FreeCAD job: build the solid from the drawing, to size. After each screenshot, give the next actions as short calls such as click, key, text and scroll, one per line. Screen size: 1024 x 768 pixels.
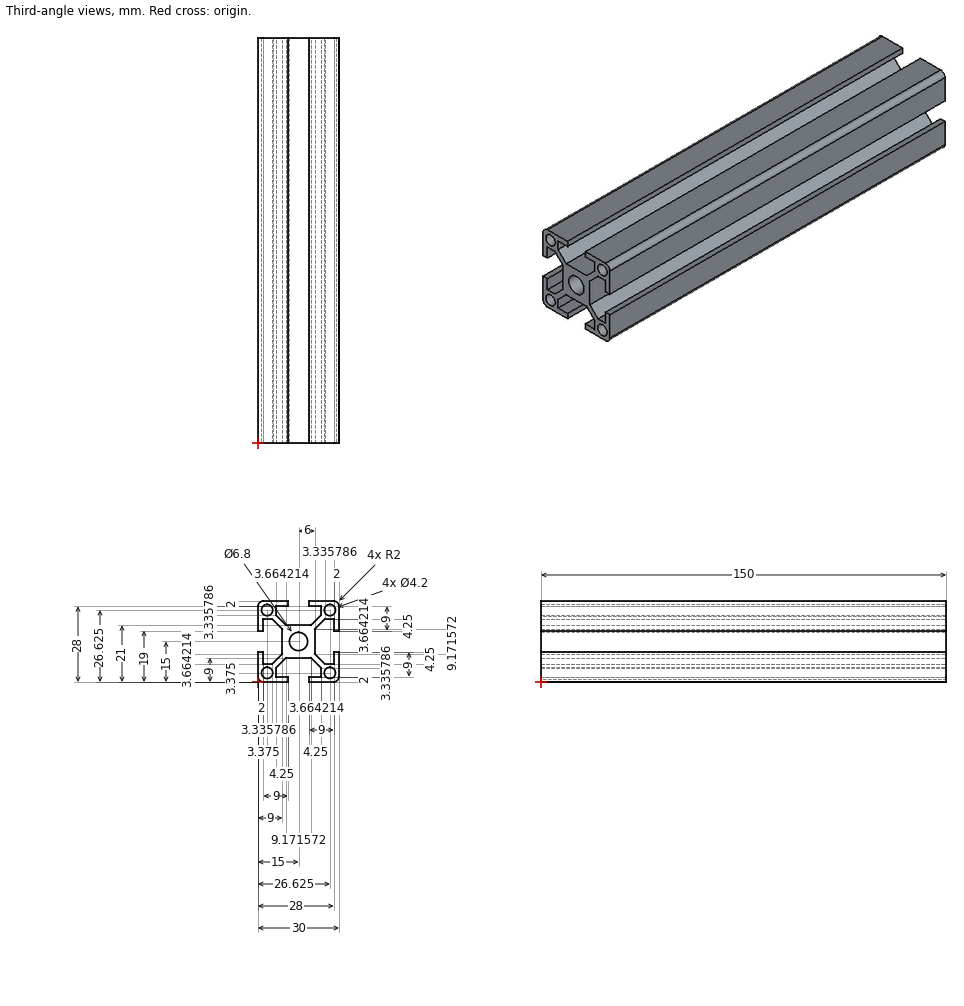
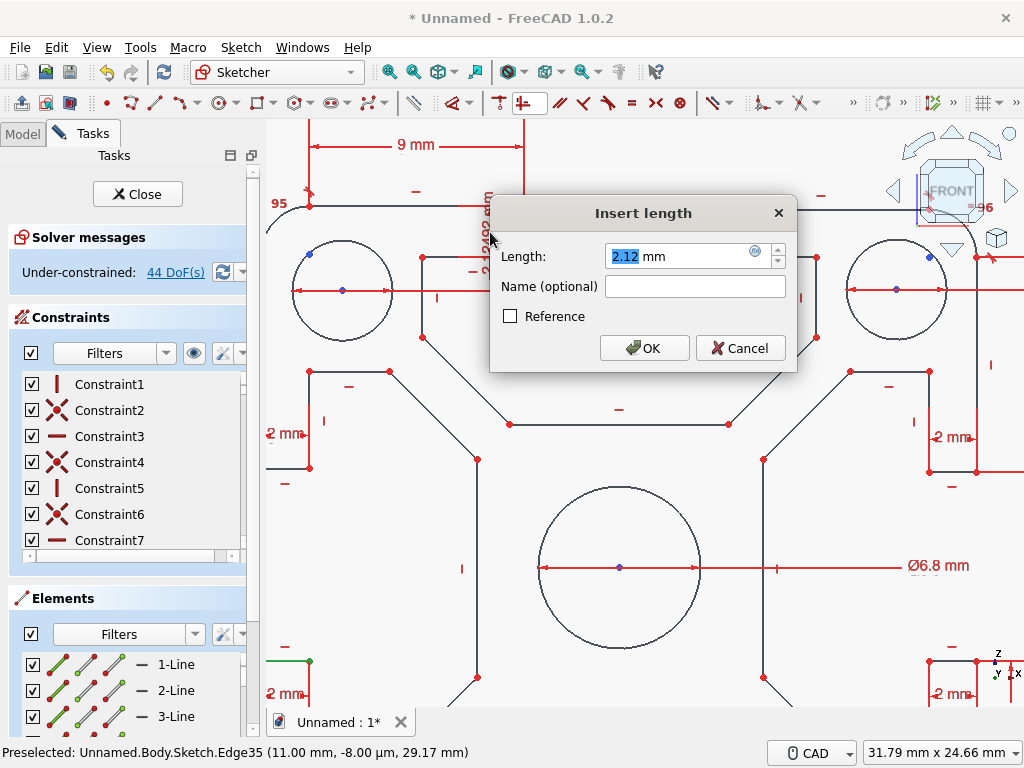
text(2)
key(Return)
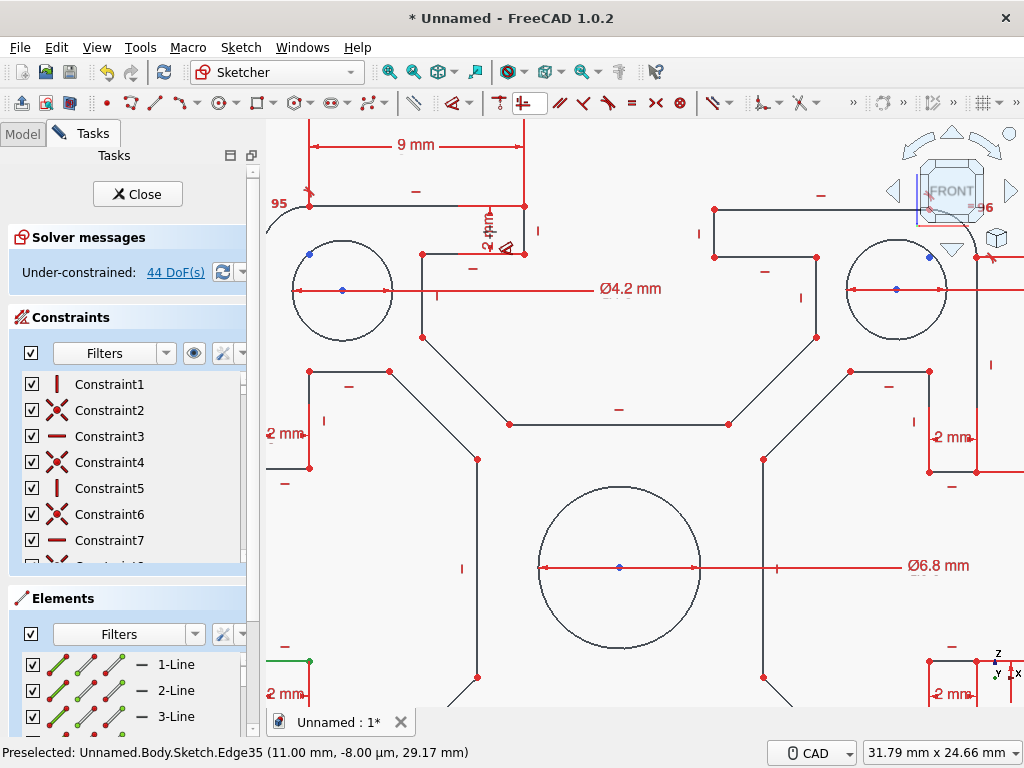
click(714, 243)
click(748, 233)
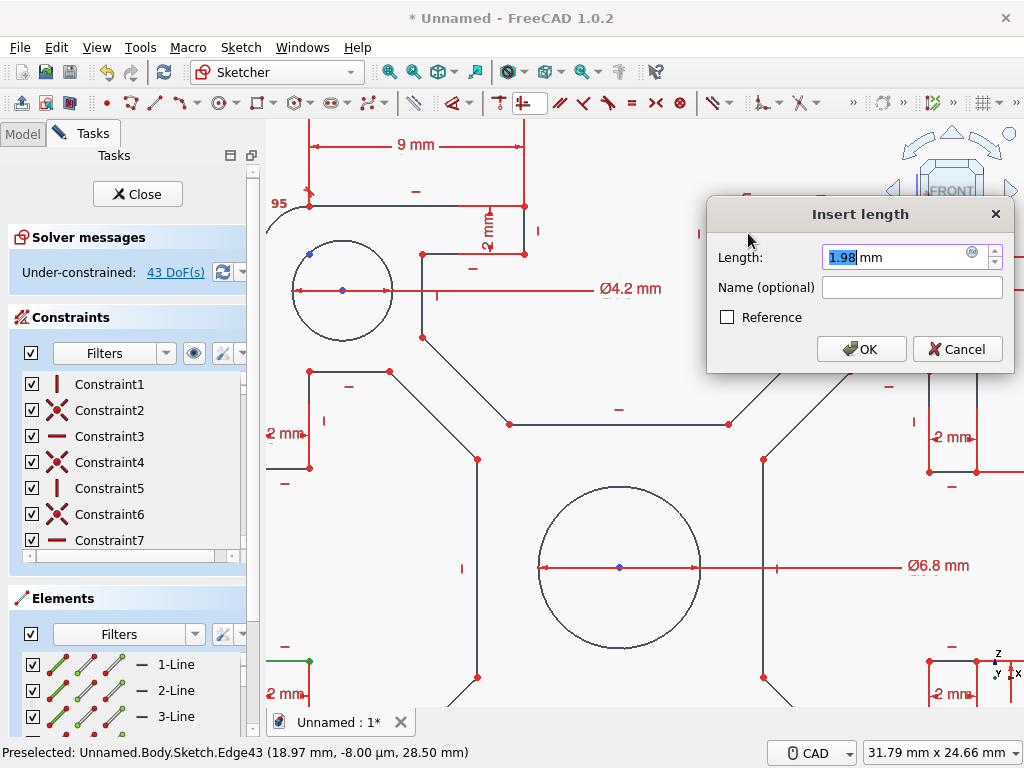
text(2)
key(Return)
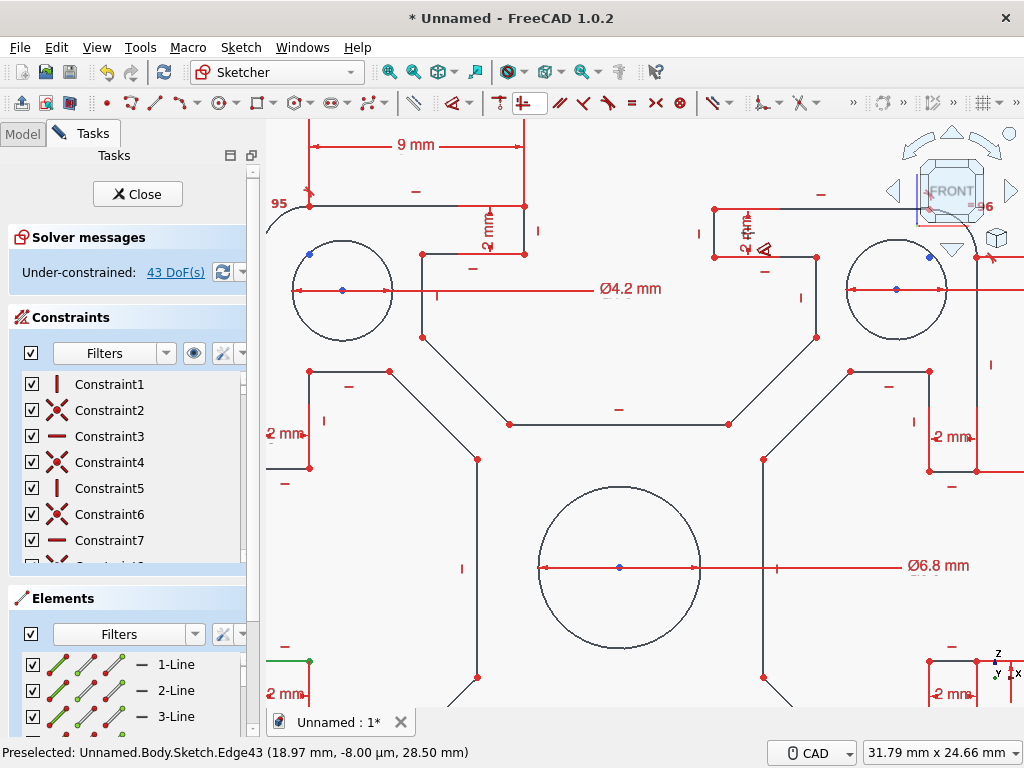
click(779, 209)
click(787, 175)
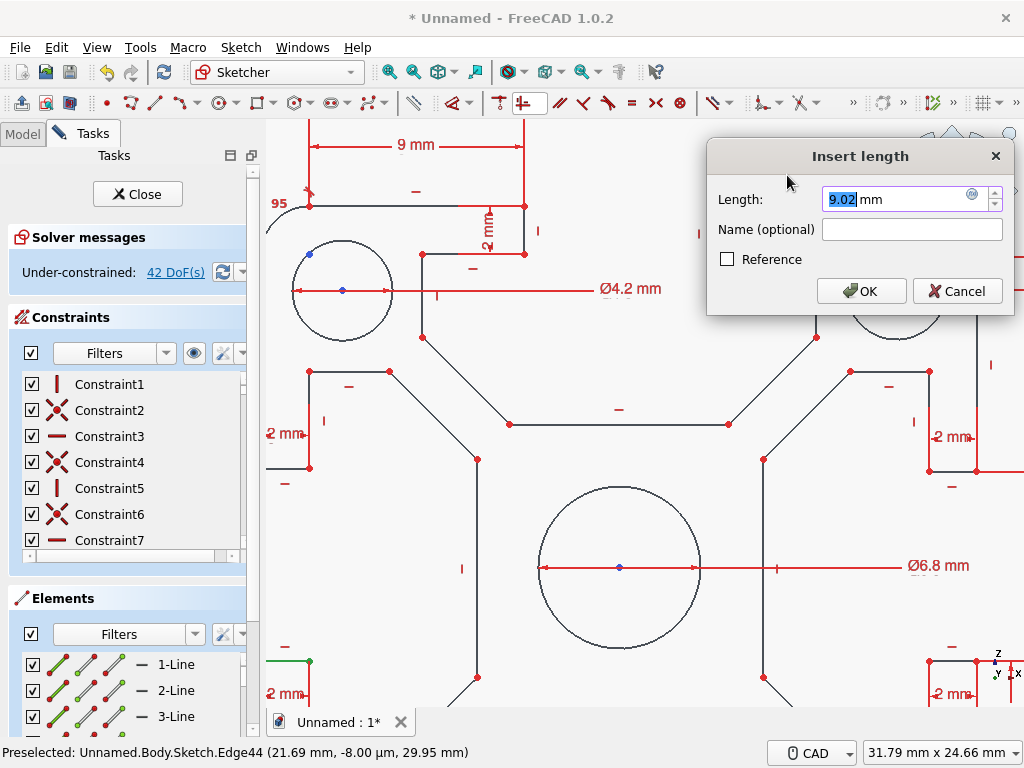
text(9)
key(Return)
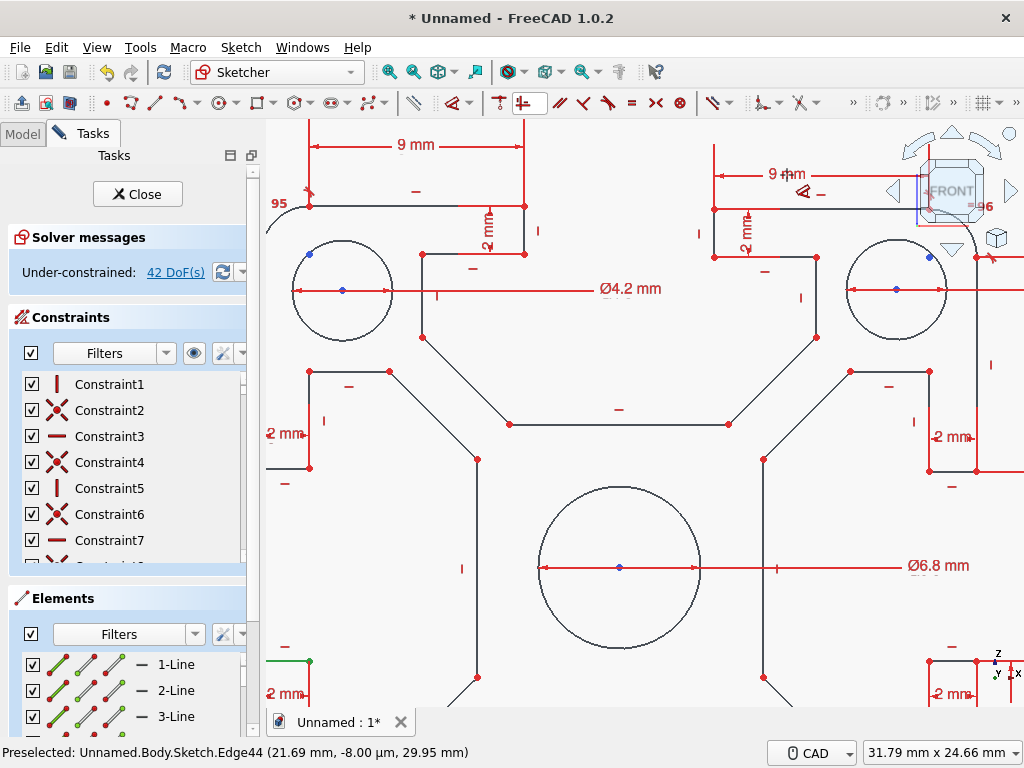
scroll(524, 227, down, 3)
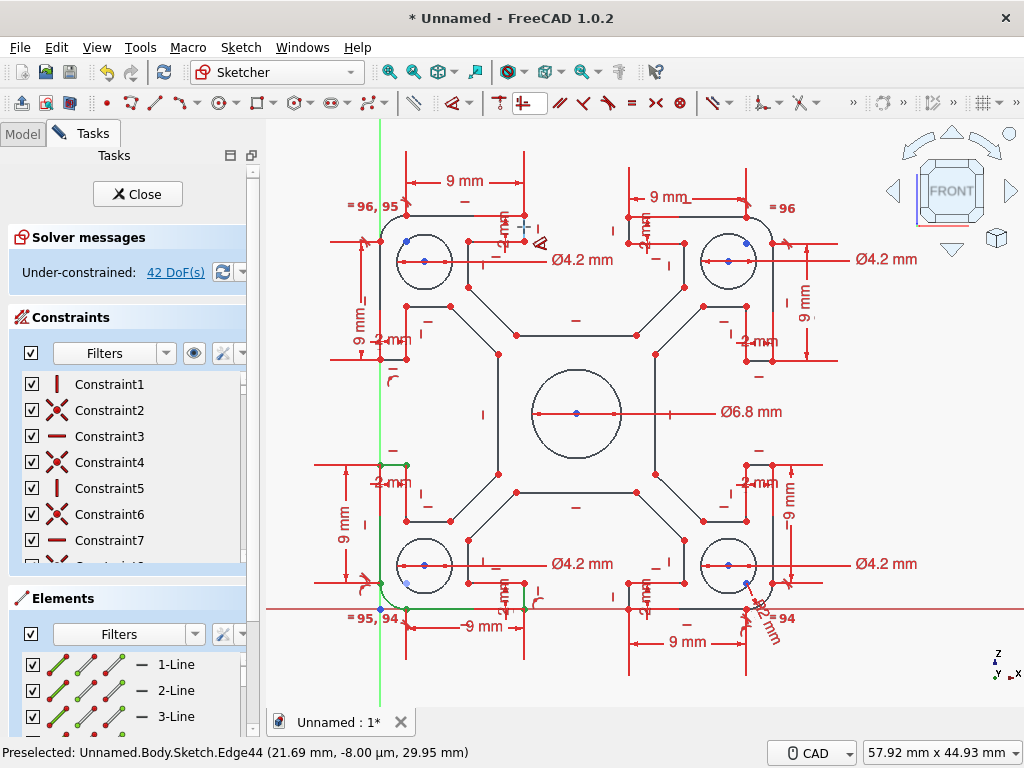
click(636, 493)
click(346, 551)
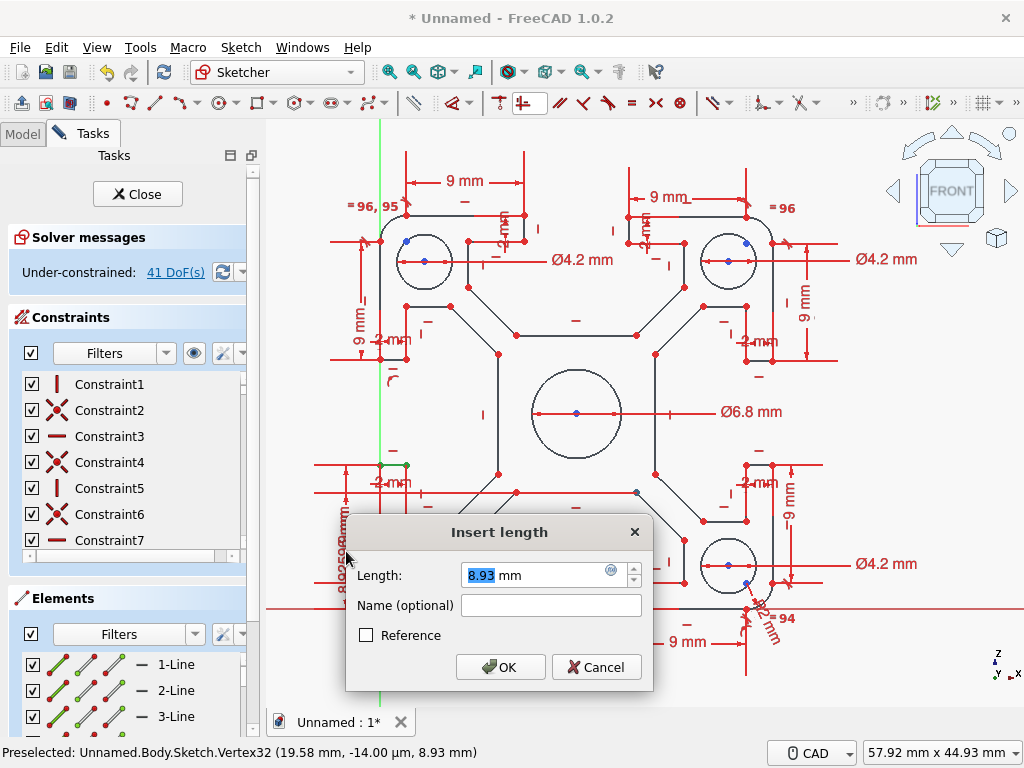
text(9)
key(Return)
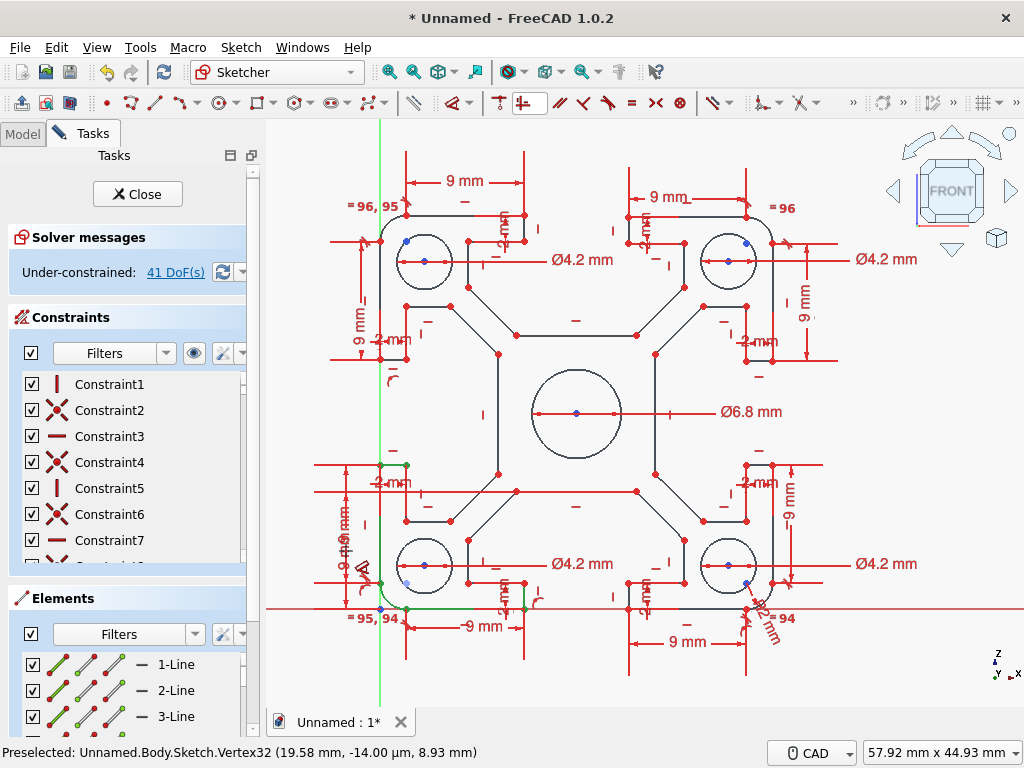
click(498, 475)
click(412, 643)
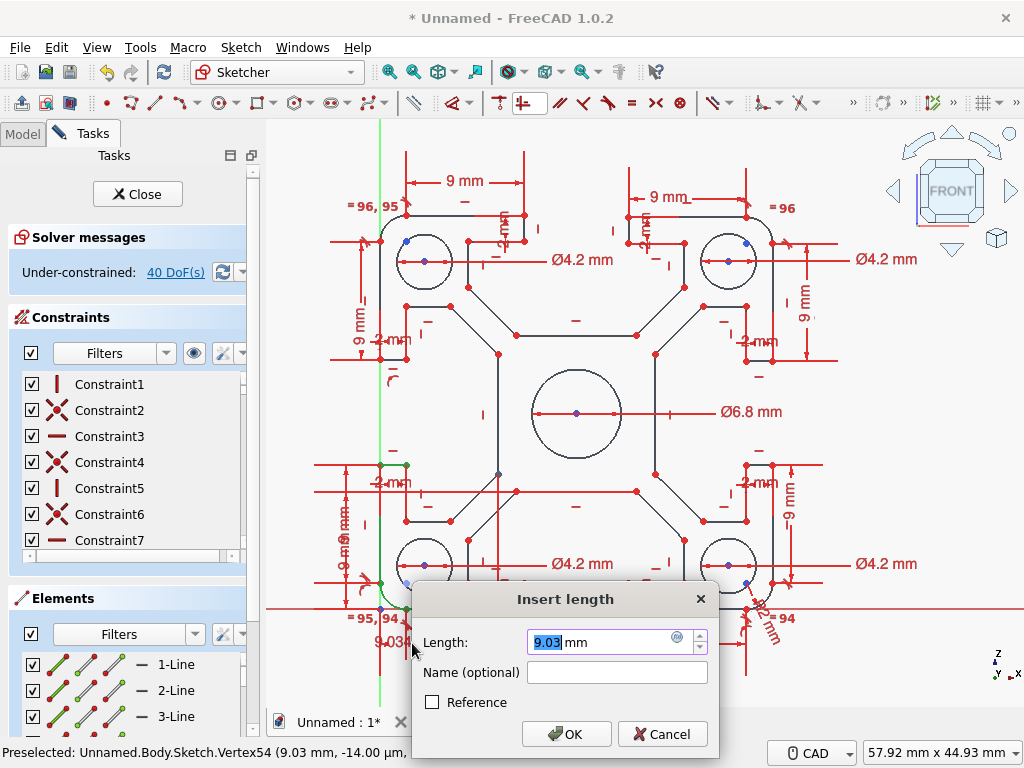
text(9)
key(Return)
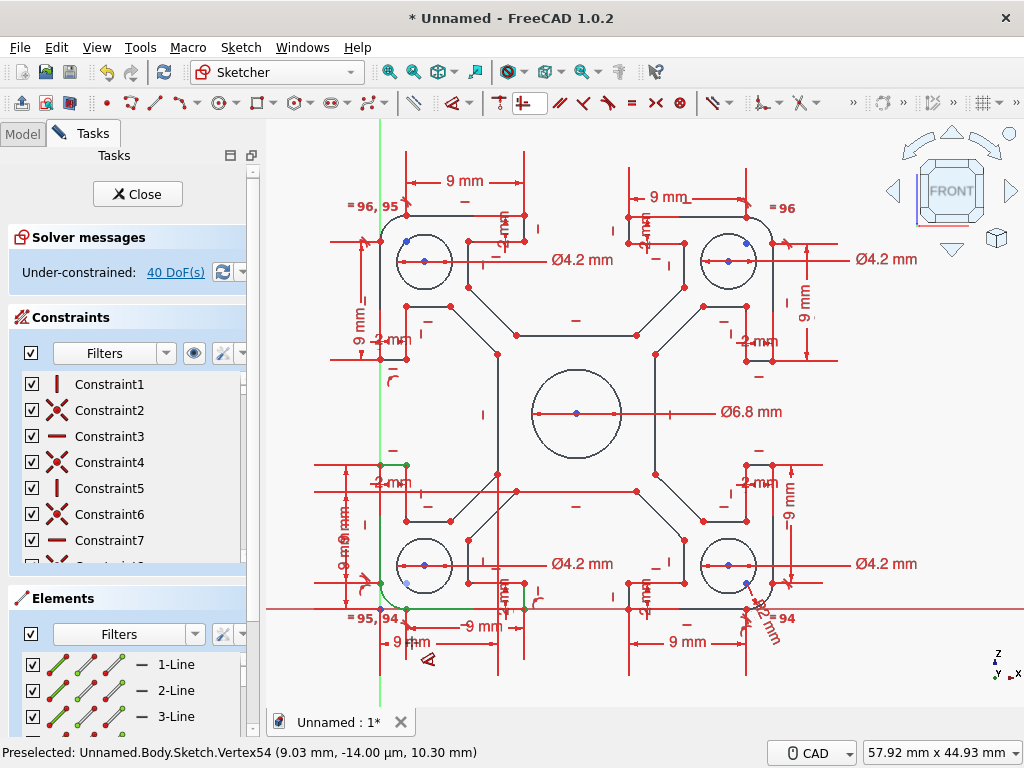
click(577, 414)
click(478, 380)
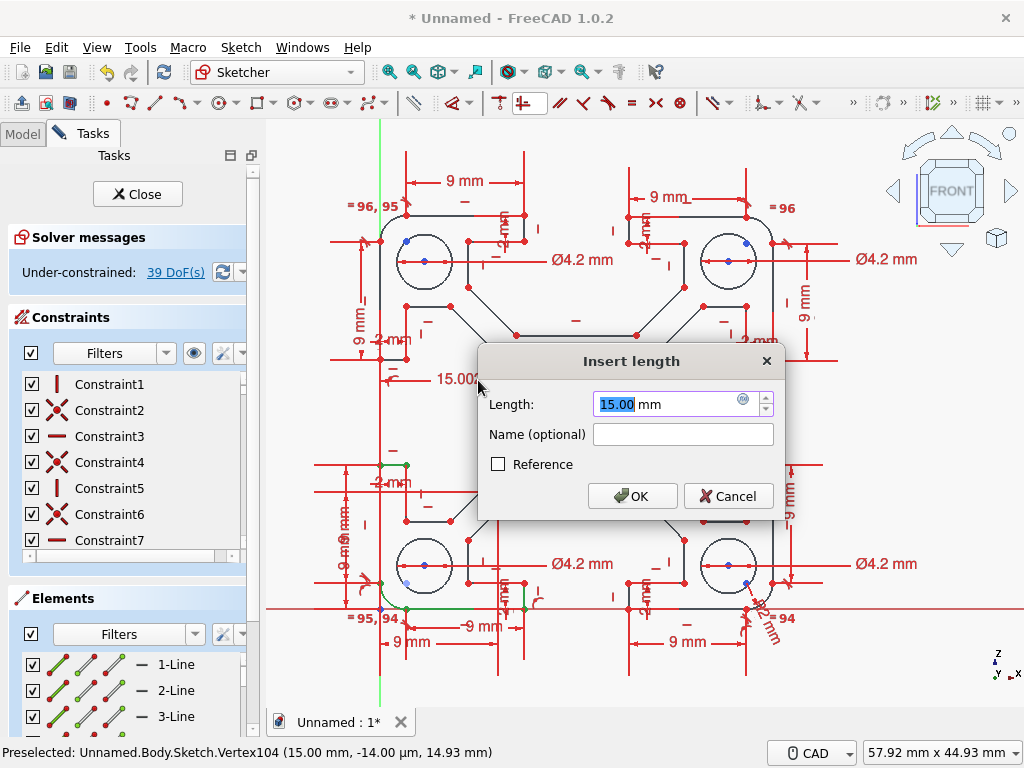
text(15)
key(Return)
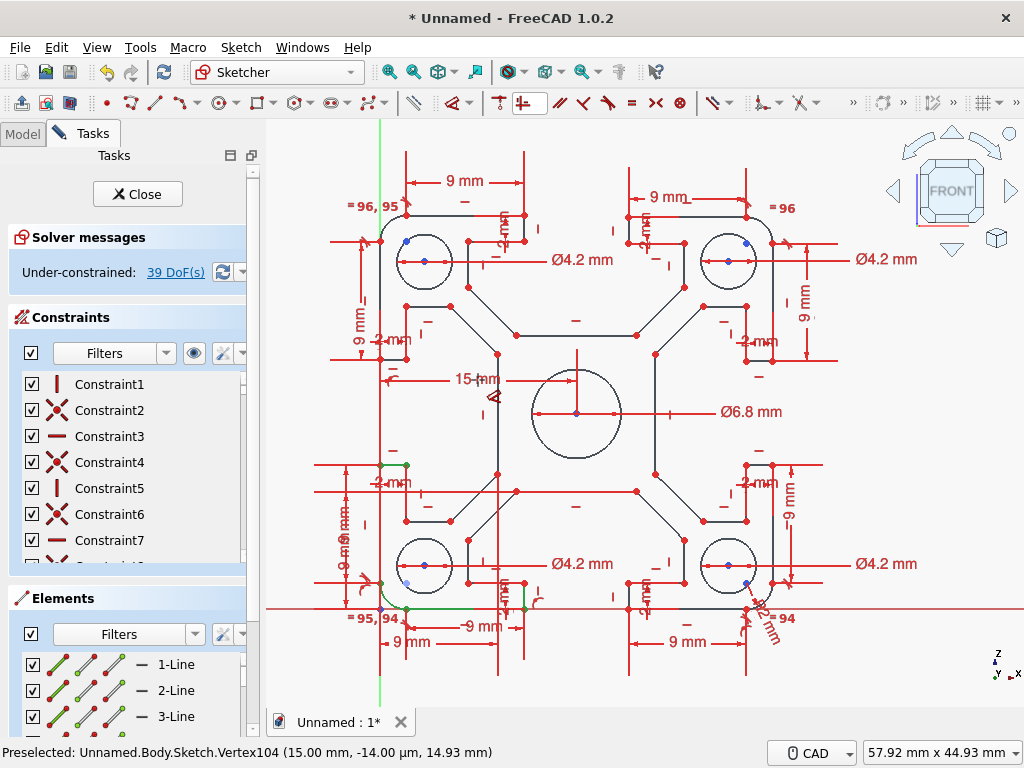
click(577, 414)
click(346, 443)